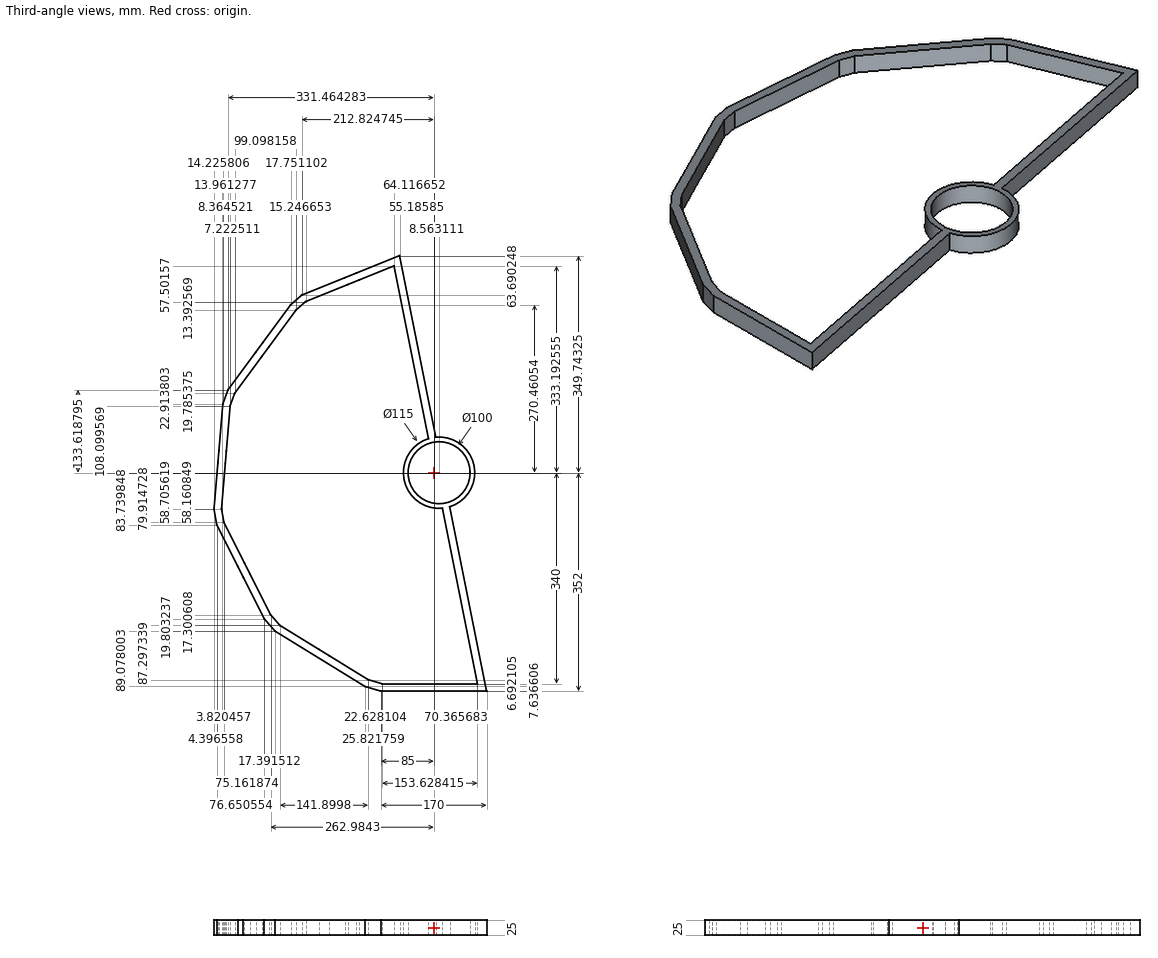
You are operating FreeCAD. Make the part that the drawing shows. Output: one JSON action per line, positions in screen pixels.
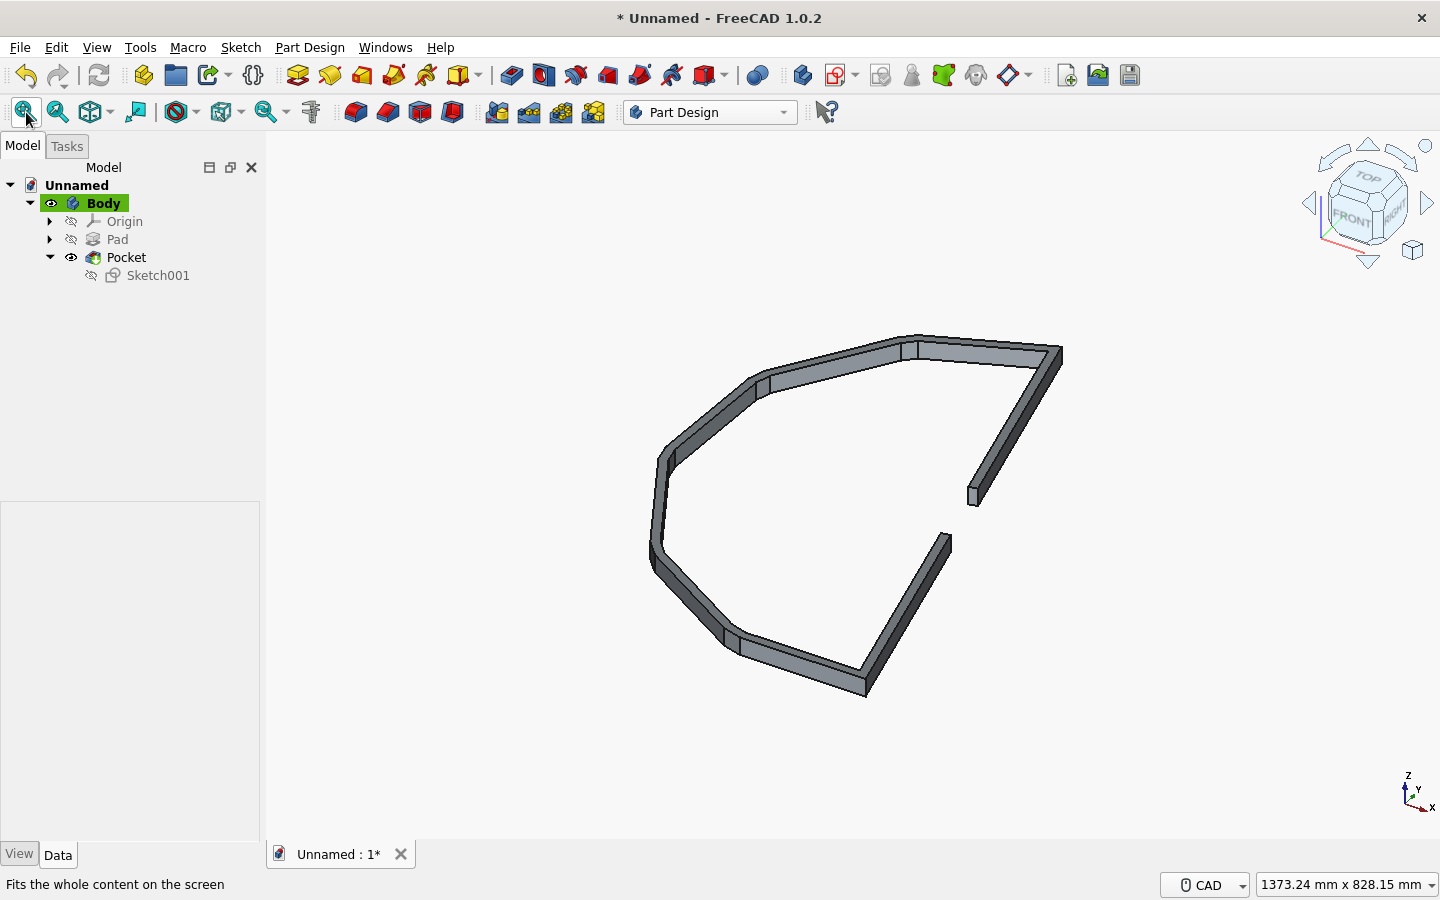
{"action": "scroll", "coordinate": [999, 442], "scroll_direction": "up", "scroll_amount": 5}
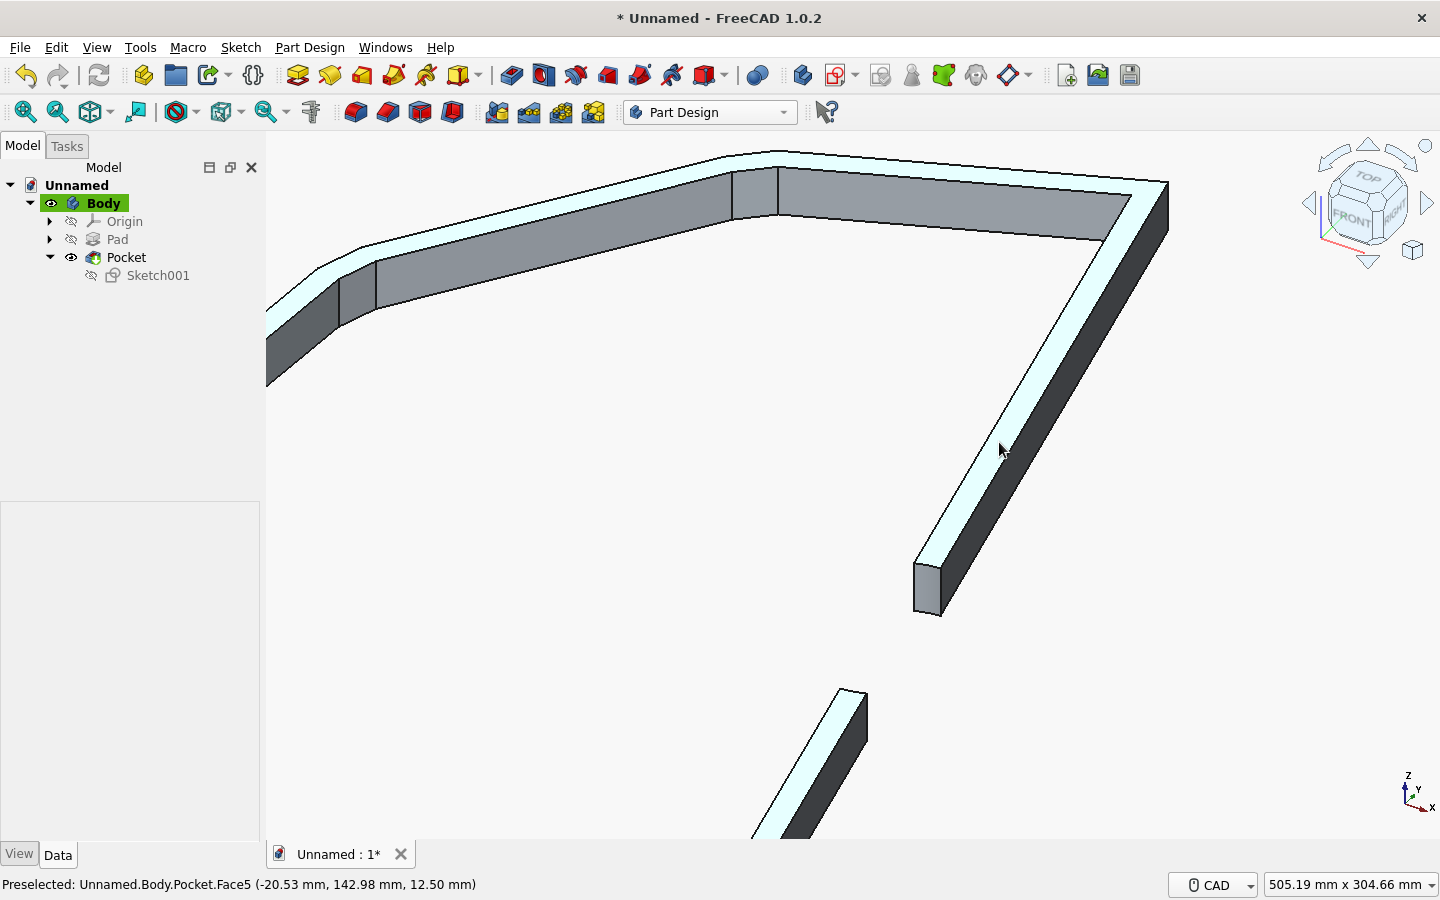
{"action": "left_click", "coordinate": [999, 442]}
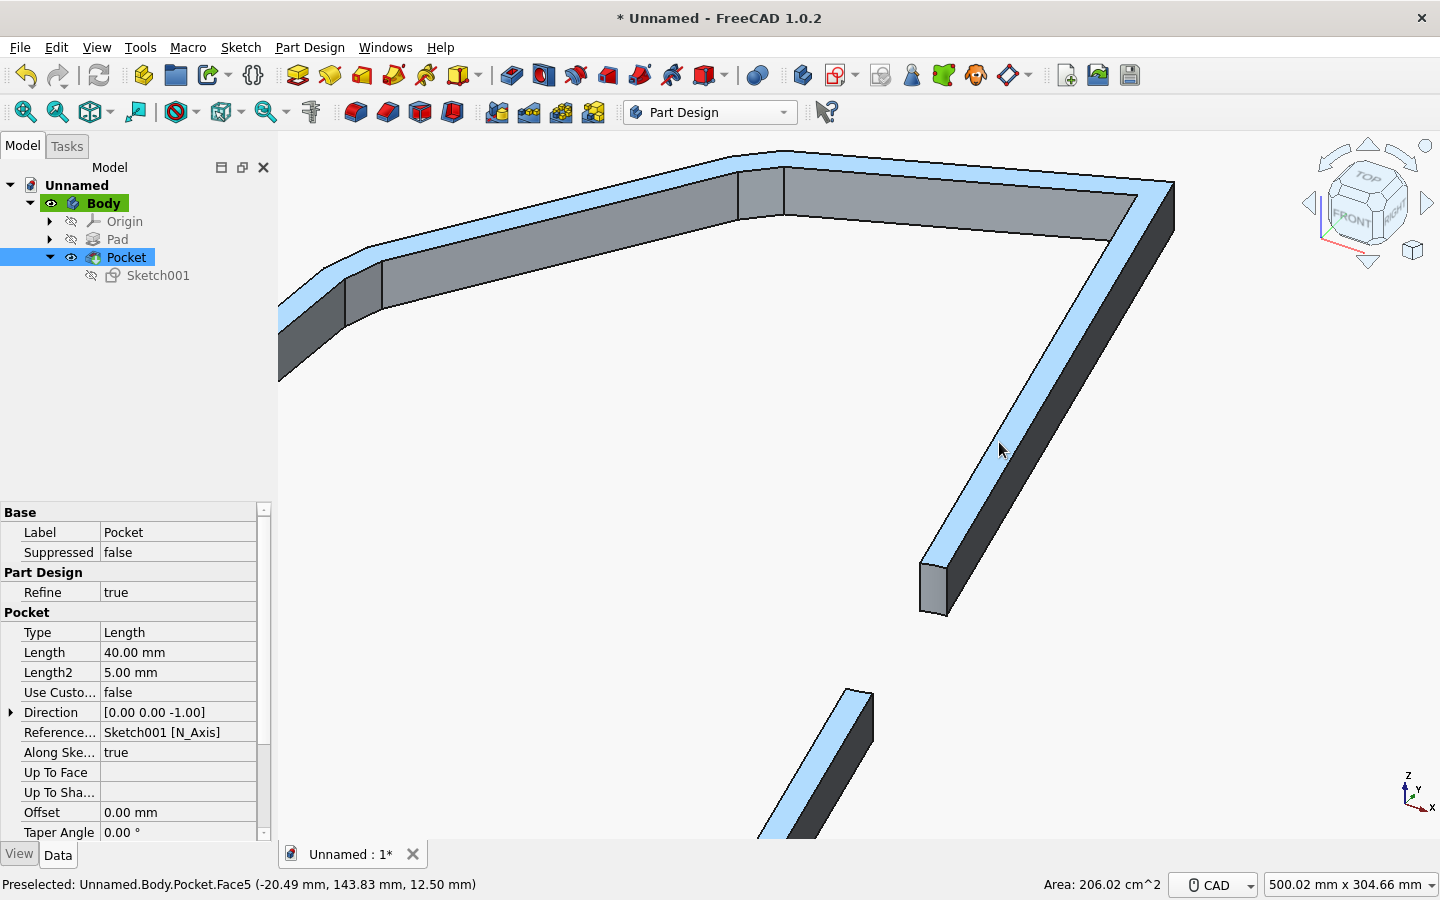
{"action": "left_click", "coordinate": [836, 76]}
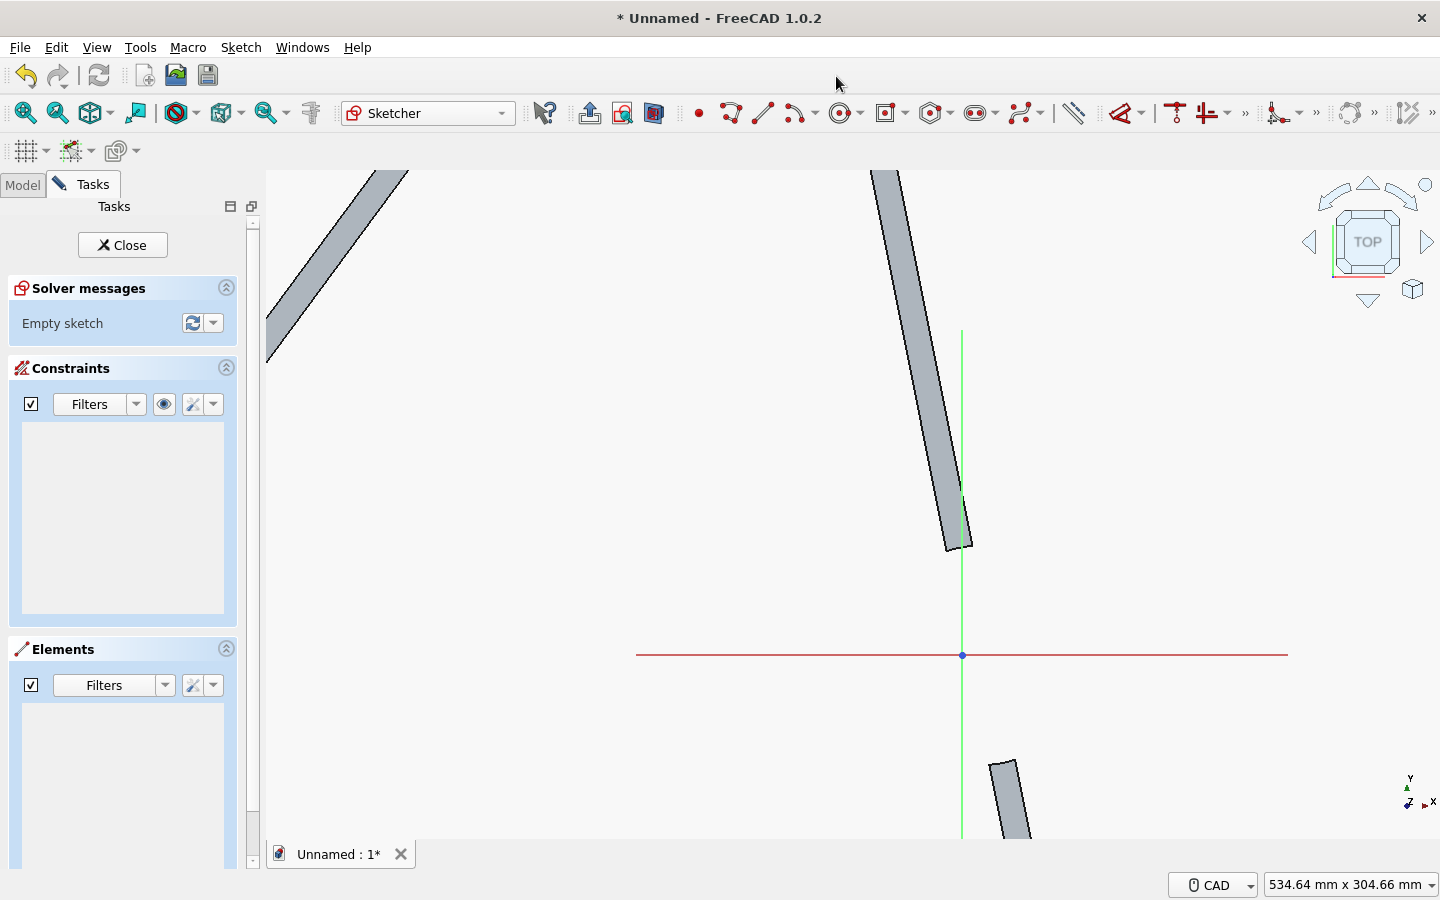
{"action": "scroll", "coordinate": [1220, 811], "scroll_direction": "up", "scroll_amount": 3}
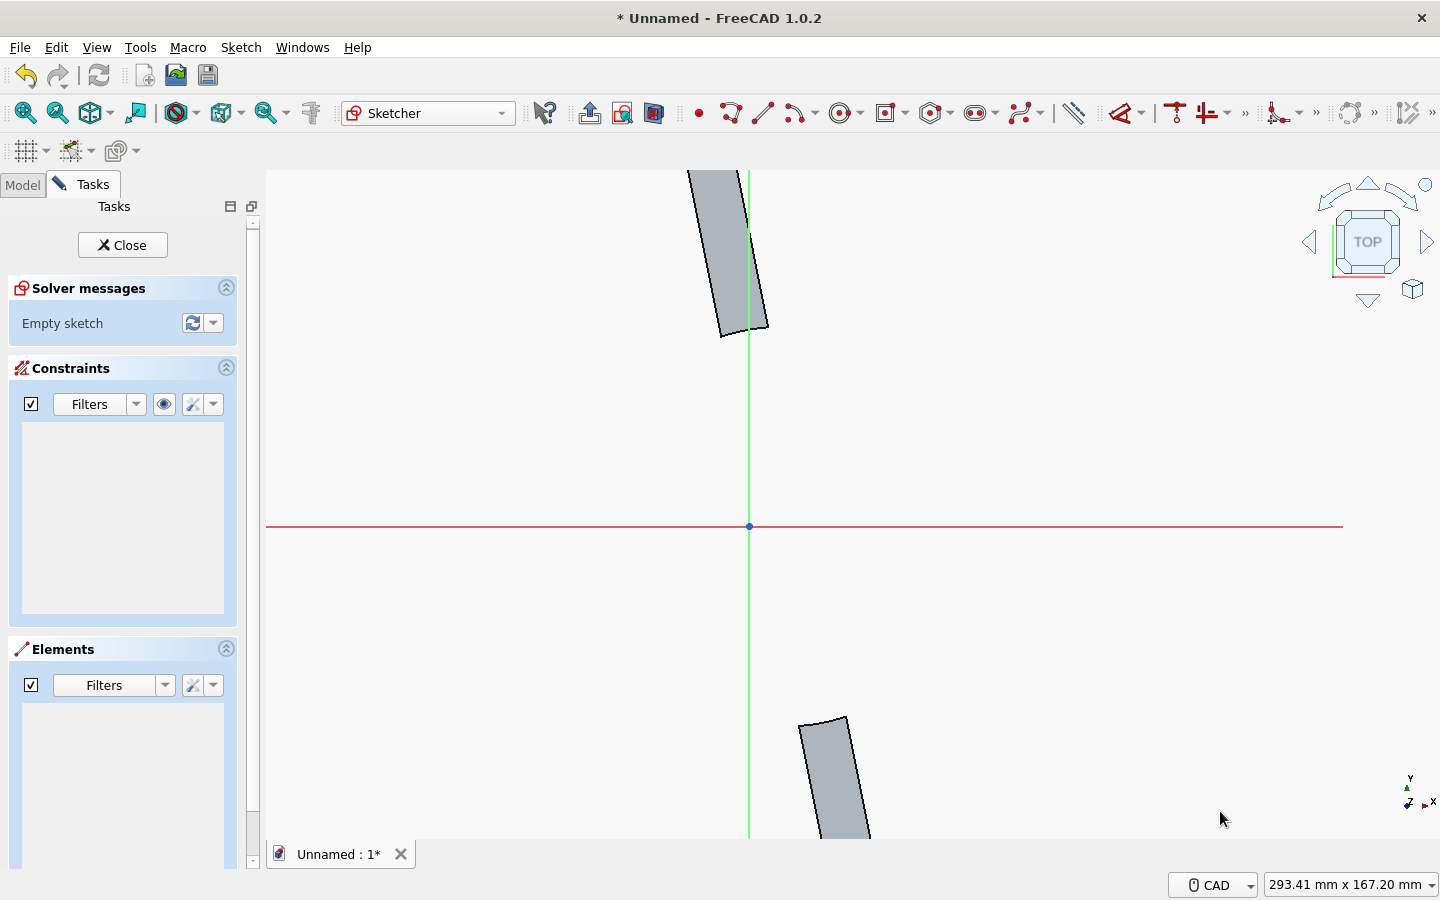
{"action": "left_click", "coordinate": [840, 114]}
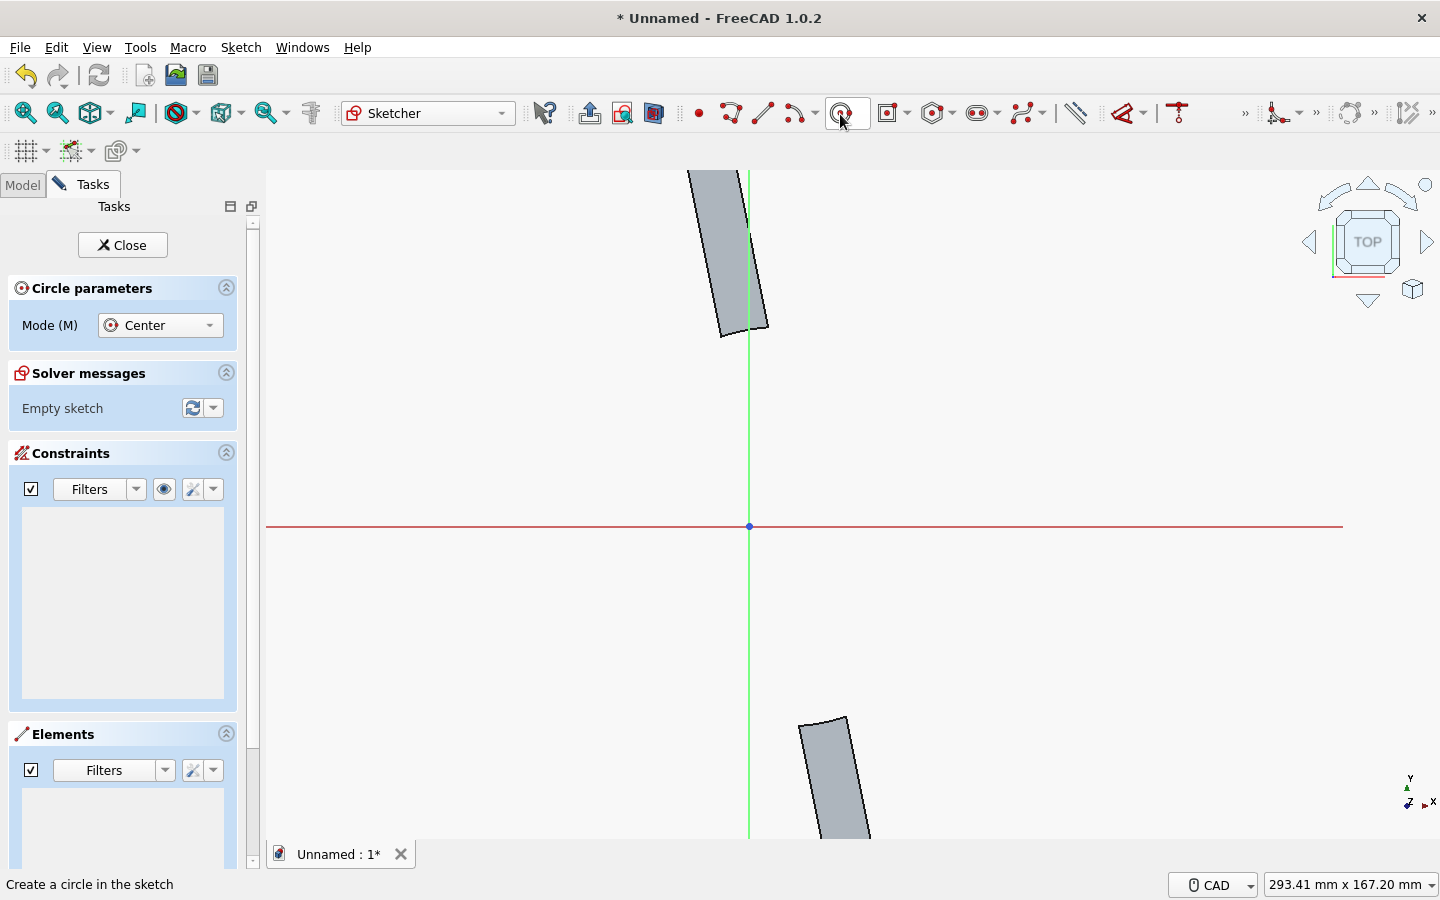
{"action": "left_click", "coordinate": [784, 527]}
{"action": "left_click", "coordinate": [946, 364]}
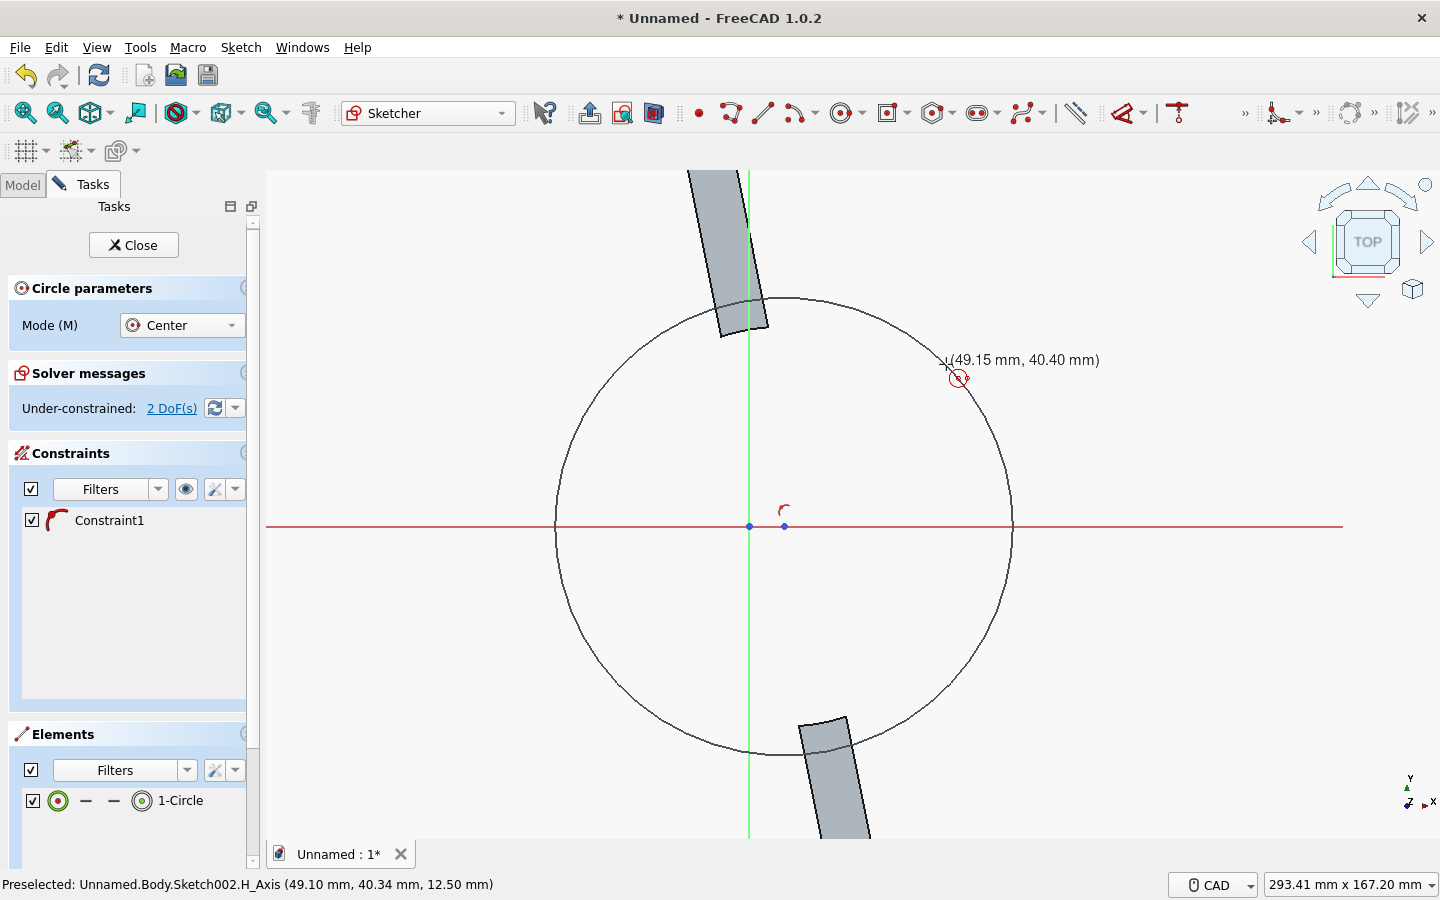
{"action": "left_click", "coordinate": [784, 527]}
{"action": "left_click", "coordinate": [925, 385]}
{"action": "key", "text": "Escape"}